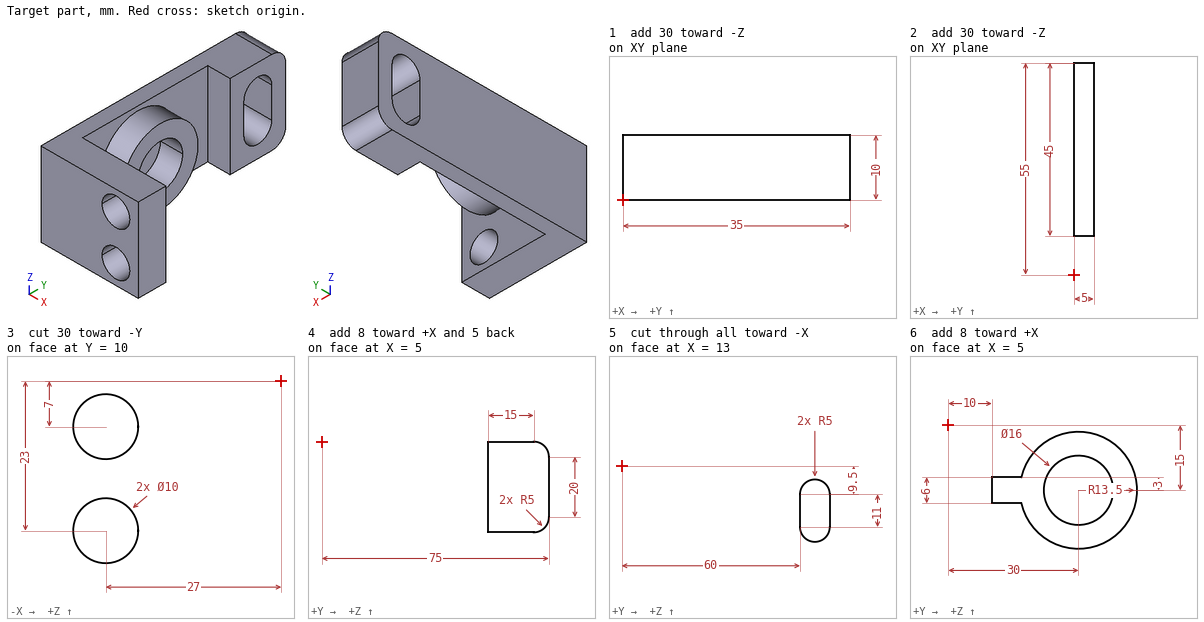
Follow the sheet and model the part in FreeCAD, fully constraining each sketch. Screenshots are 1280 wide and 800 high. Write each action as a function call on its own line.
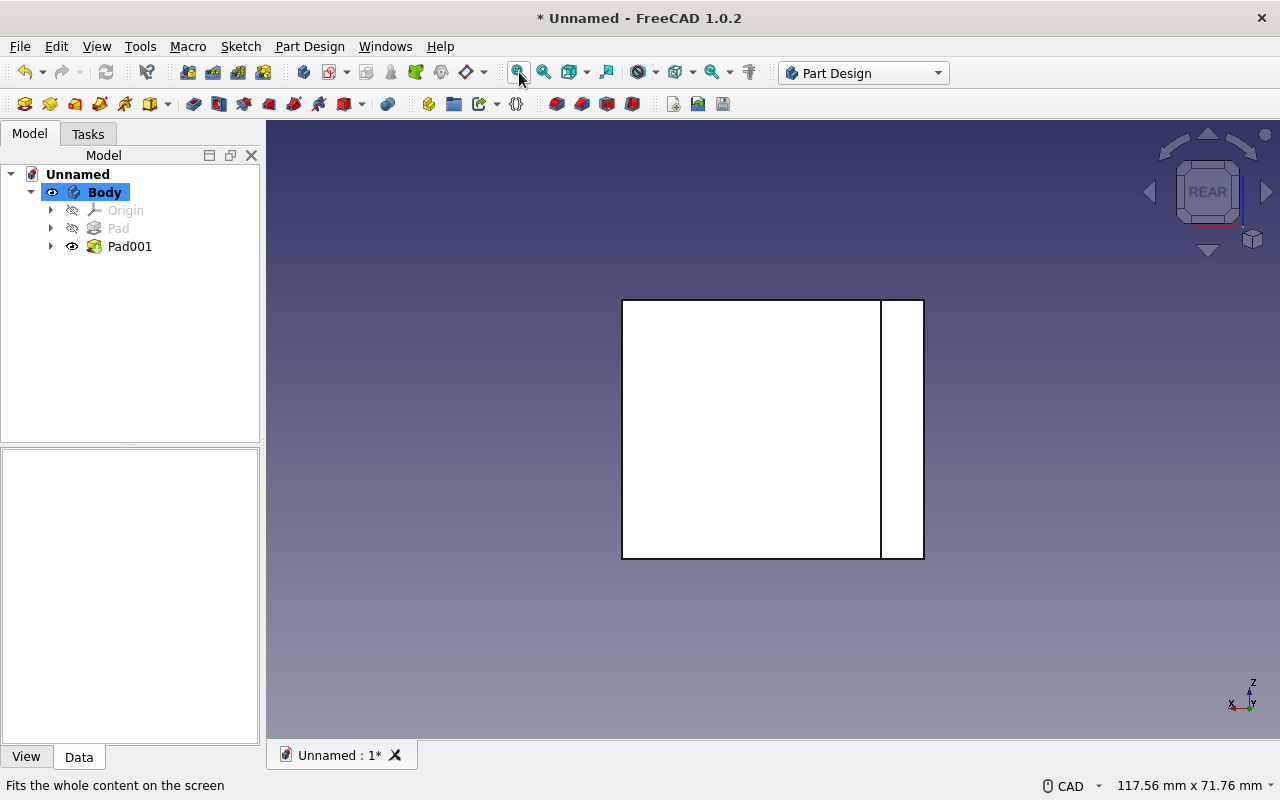
key(v)
key(f)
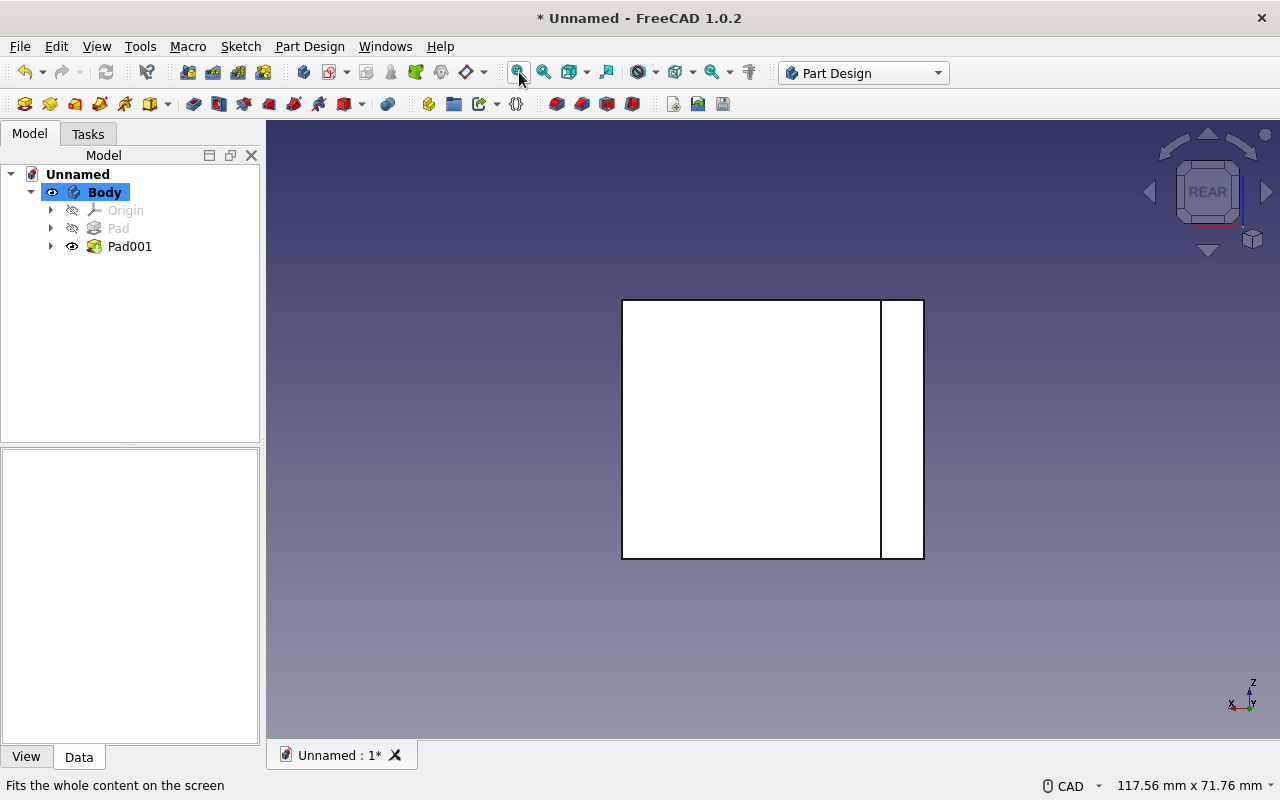
click(751, 429)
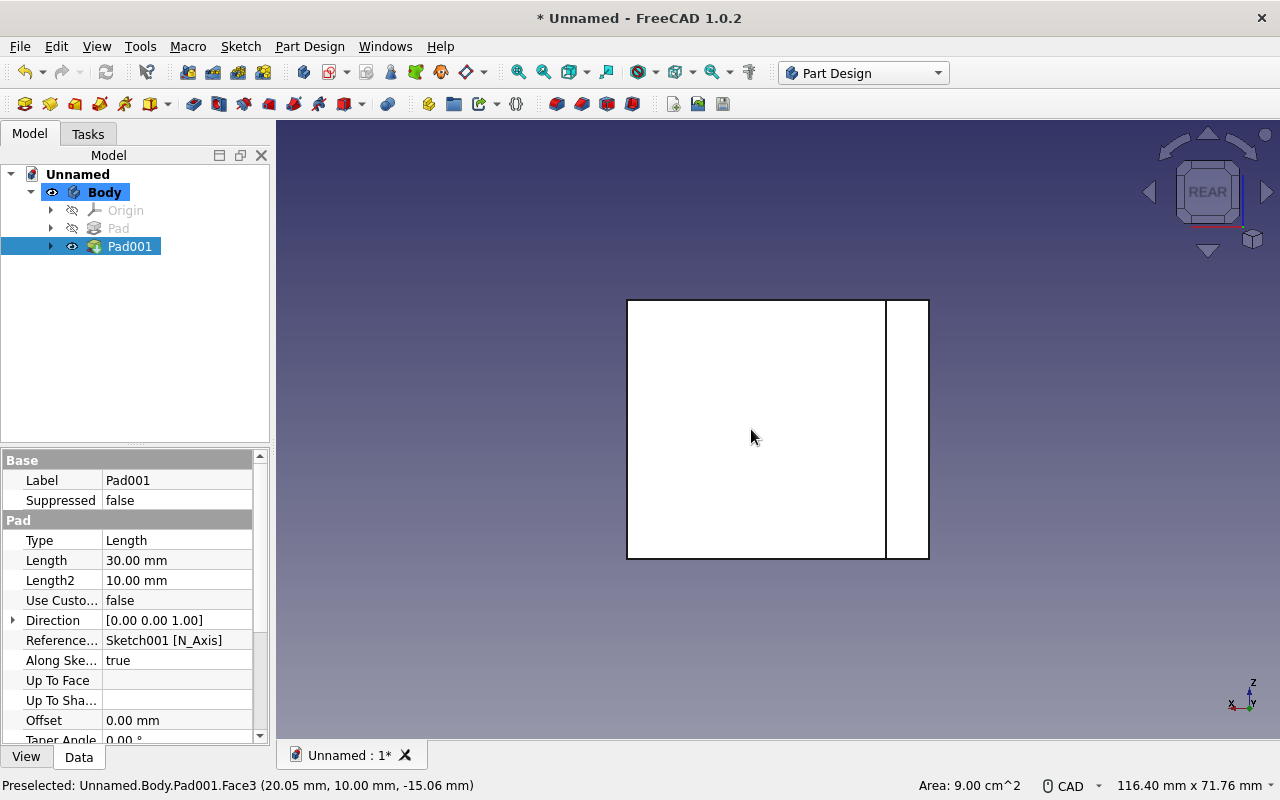
click(328, 72)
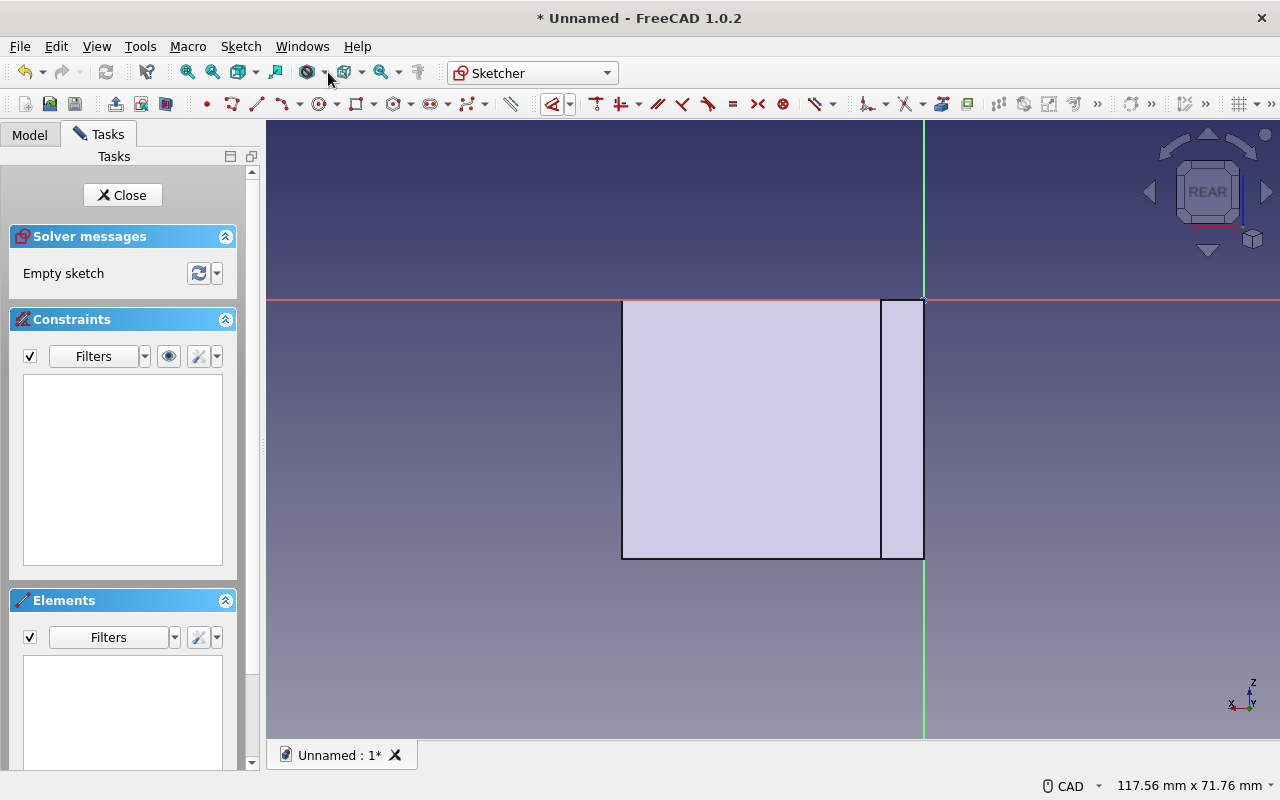
scroll(952, 403, up, 2)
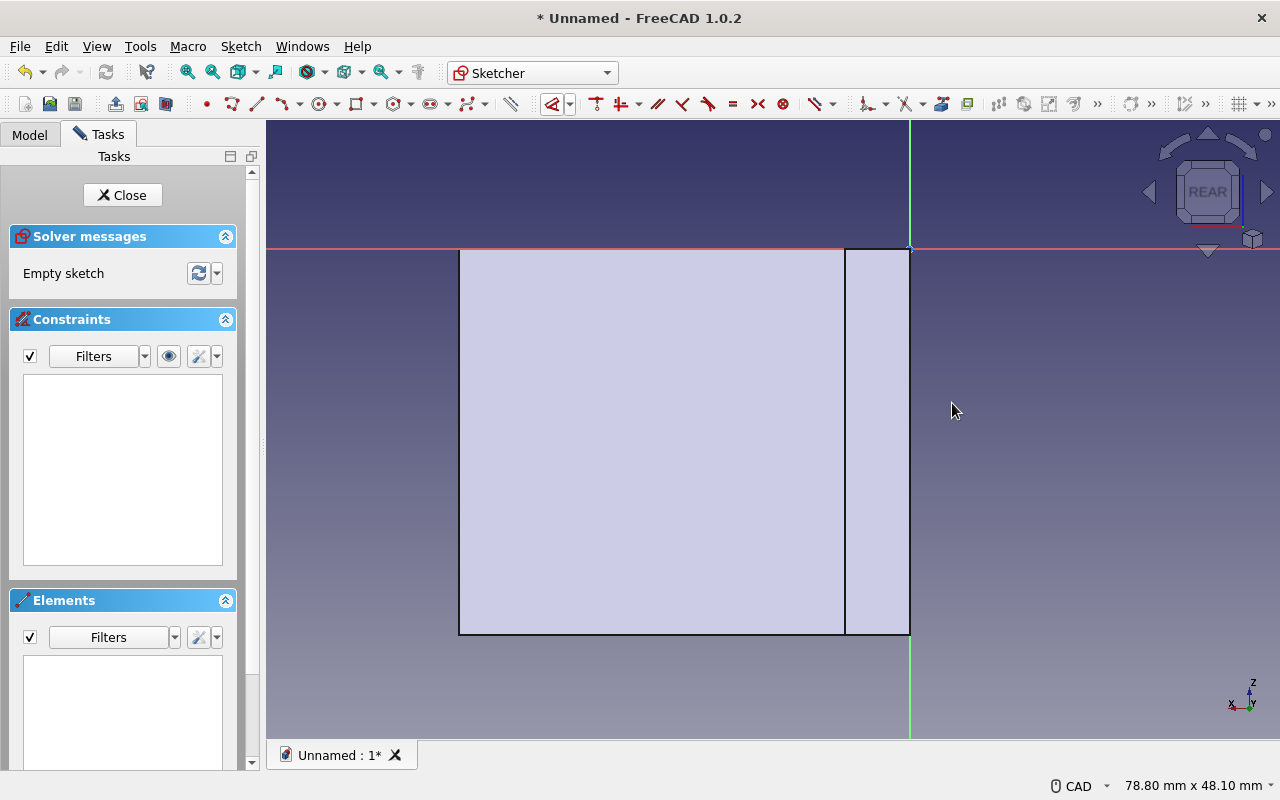
key(g)
key(c)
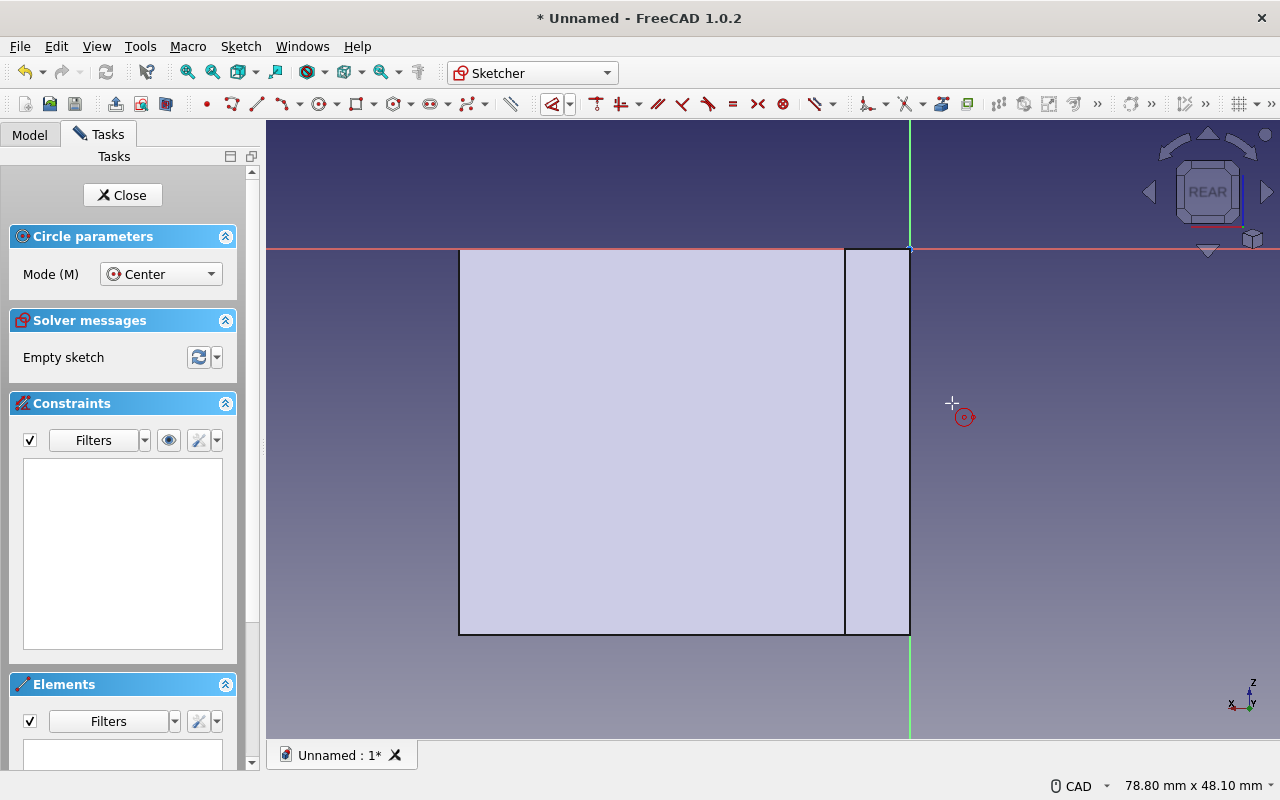
click(562, 545)
click(608, 500)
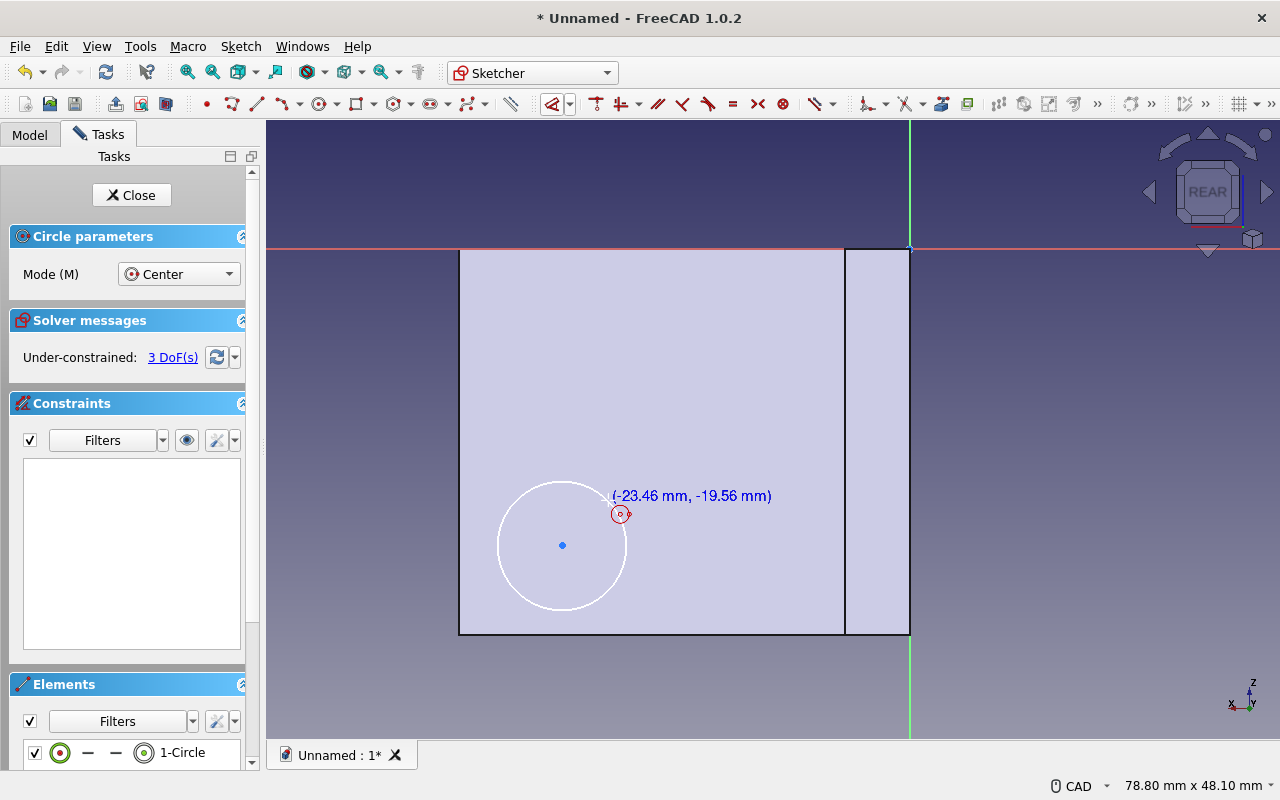
click(562, 339)
click(608, 294)
key(Escape)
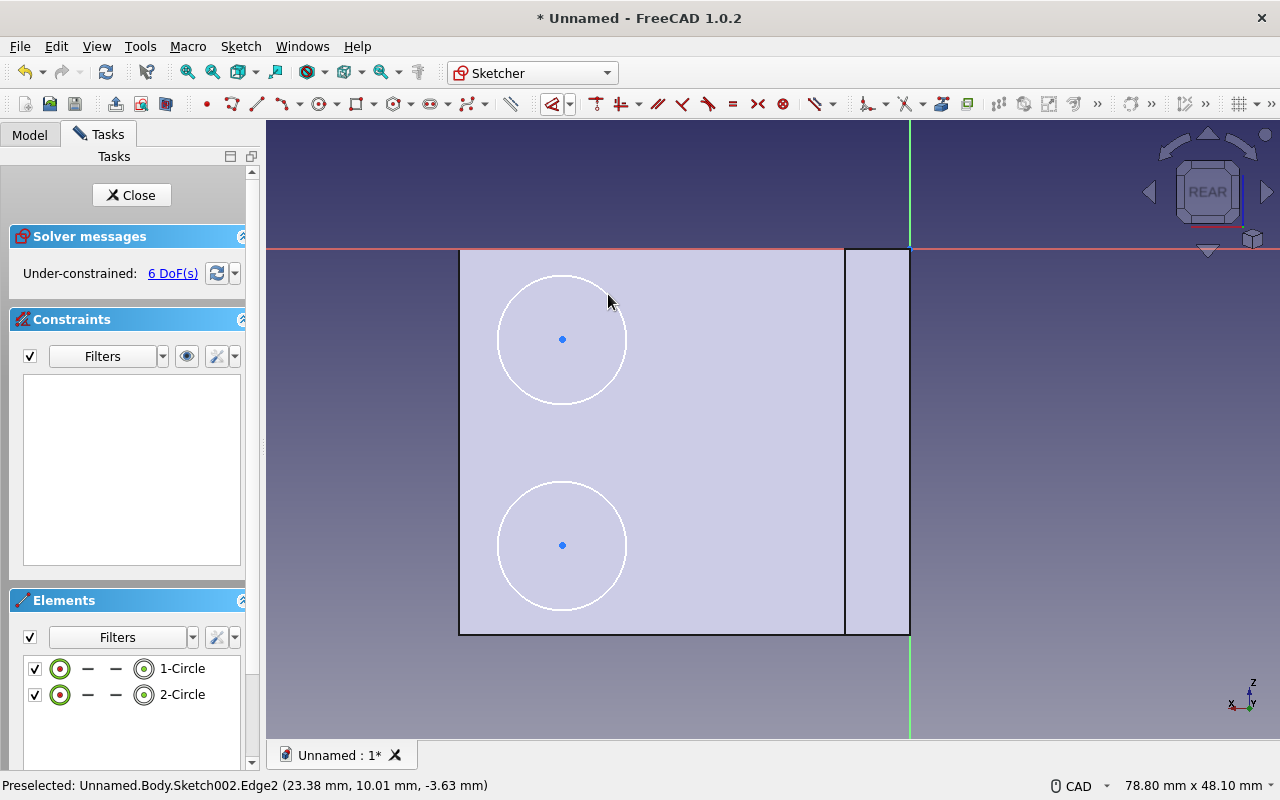
click(607, 500)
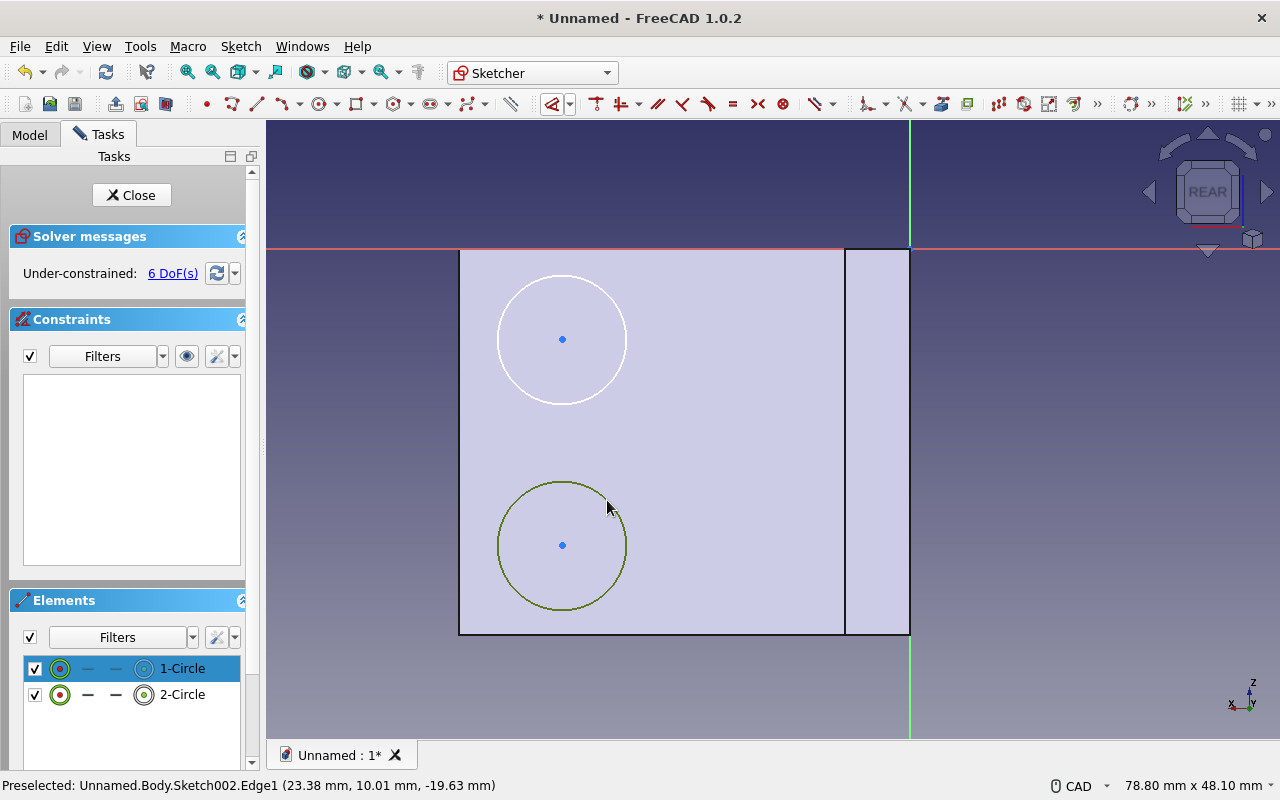
click(607, 294)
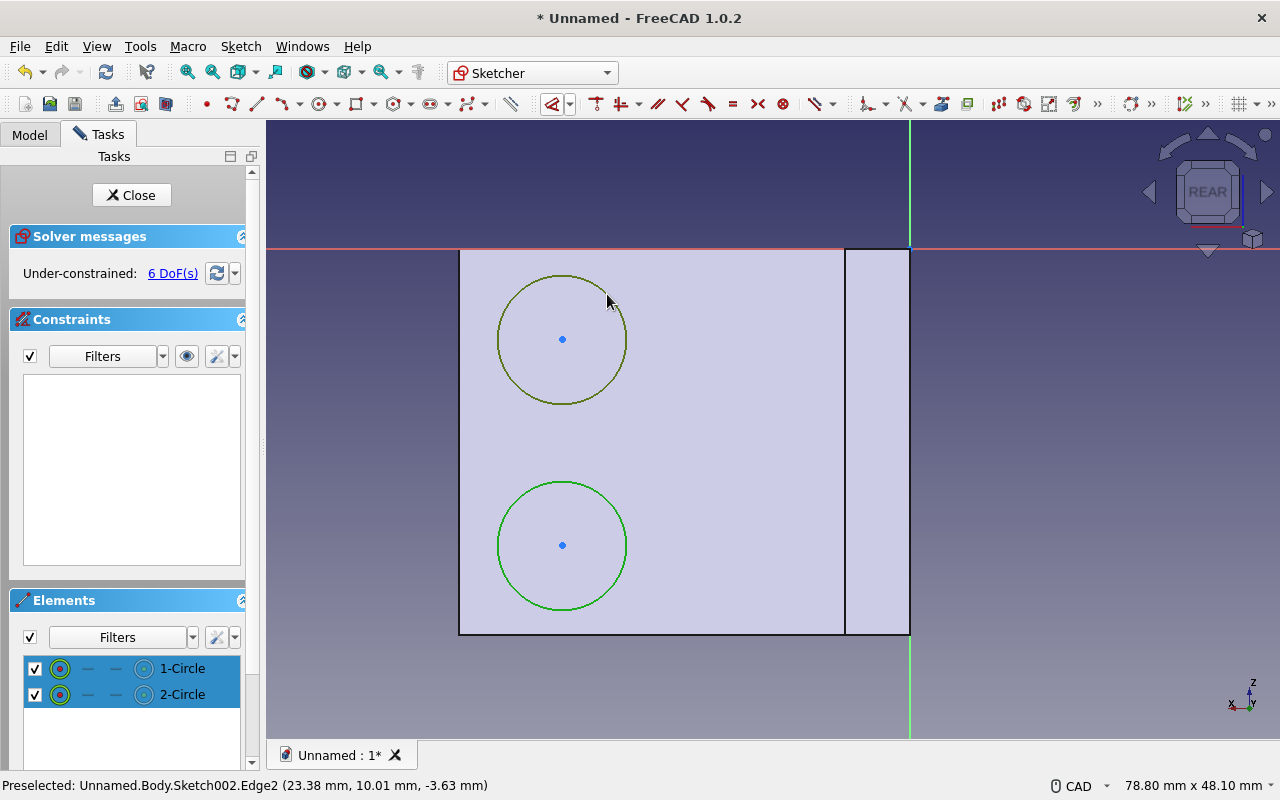
key(e)